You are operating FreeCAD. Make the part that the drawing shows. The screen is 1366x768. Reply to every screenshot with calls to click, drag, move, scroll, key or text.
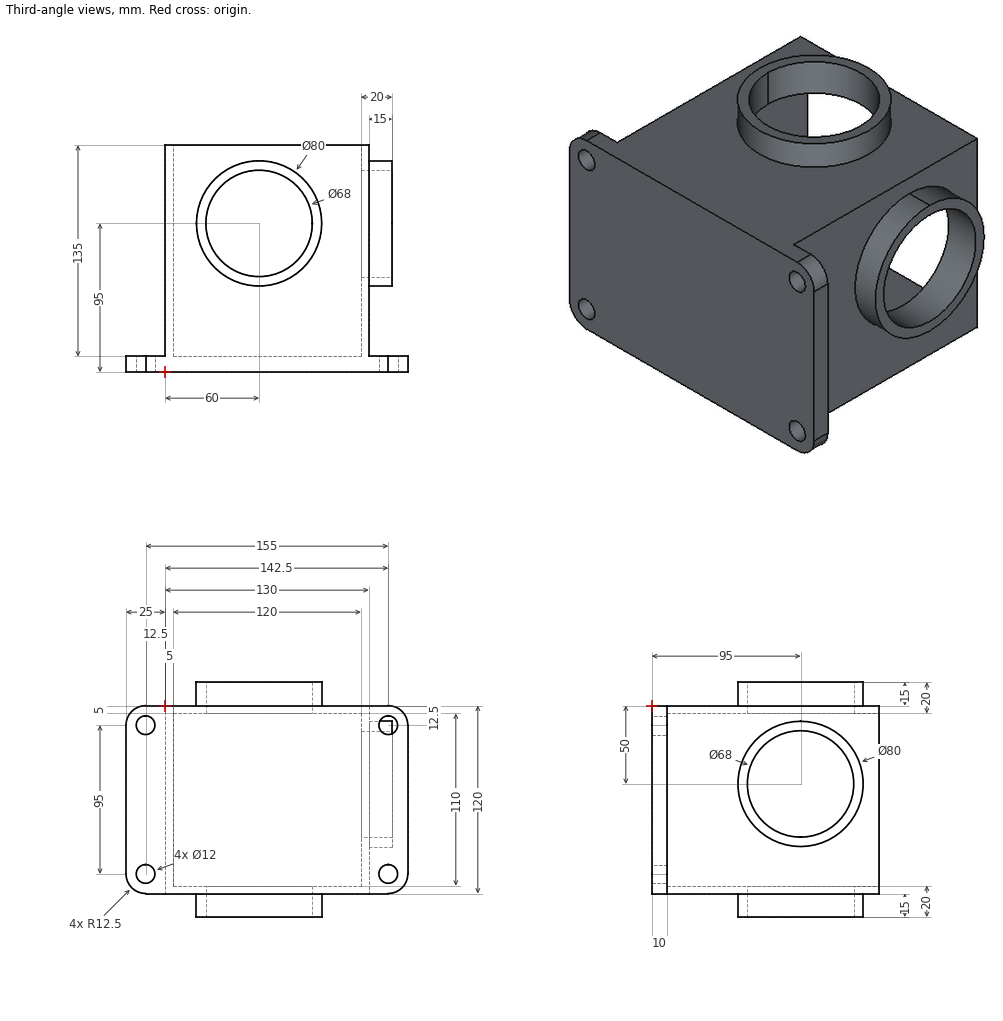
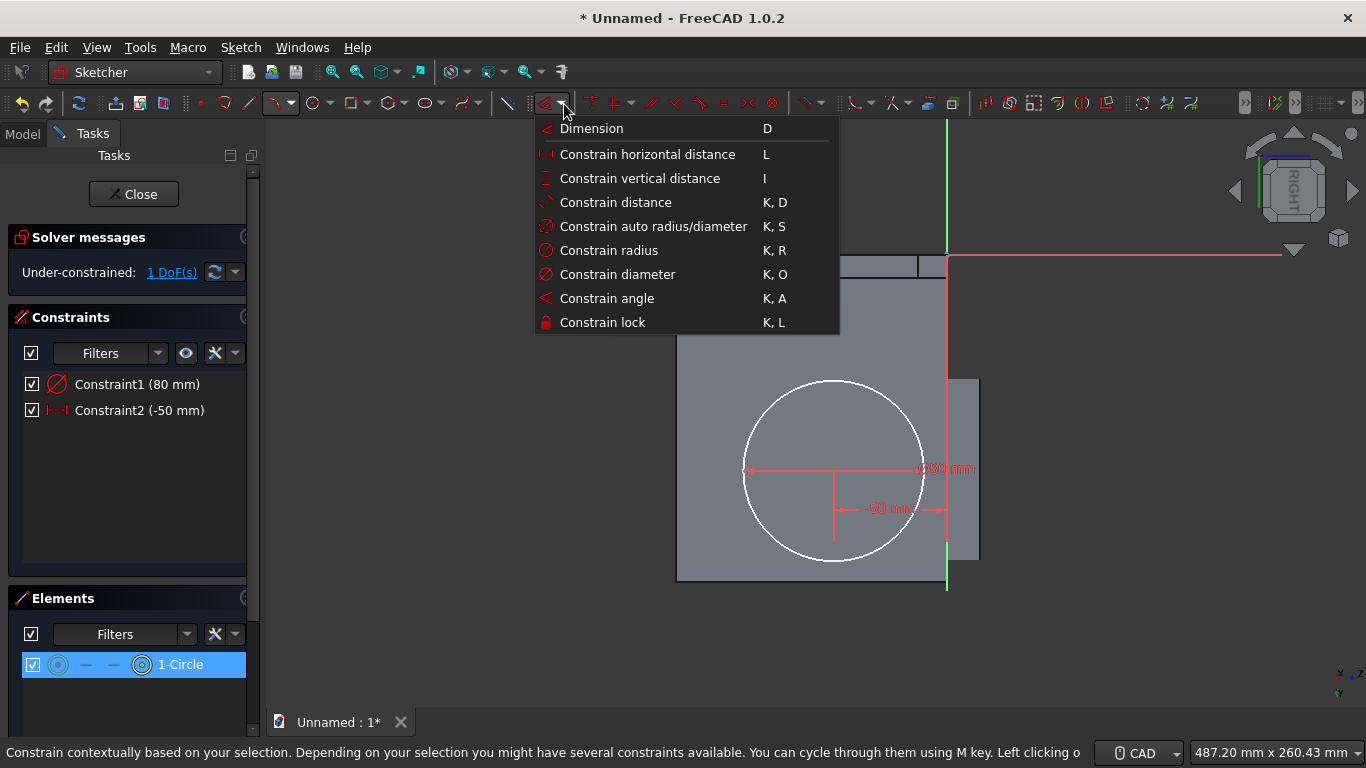
click(687, 178)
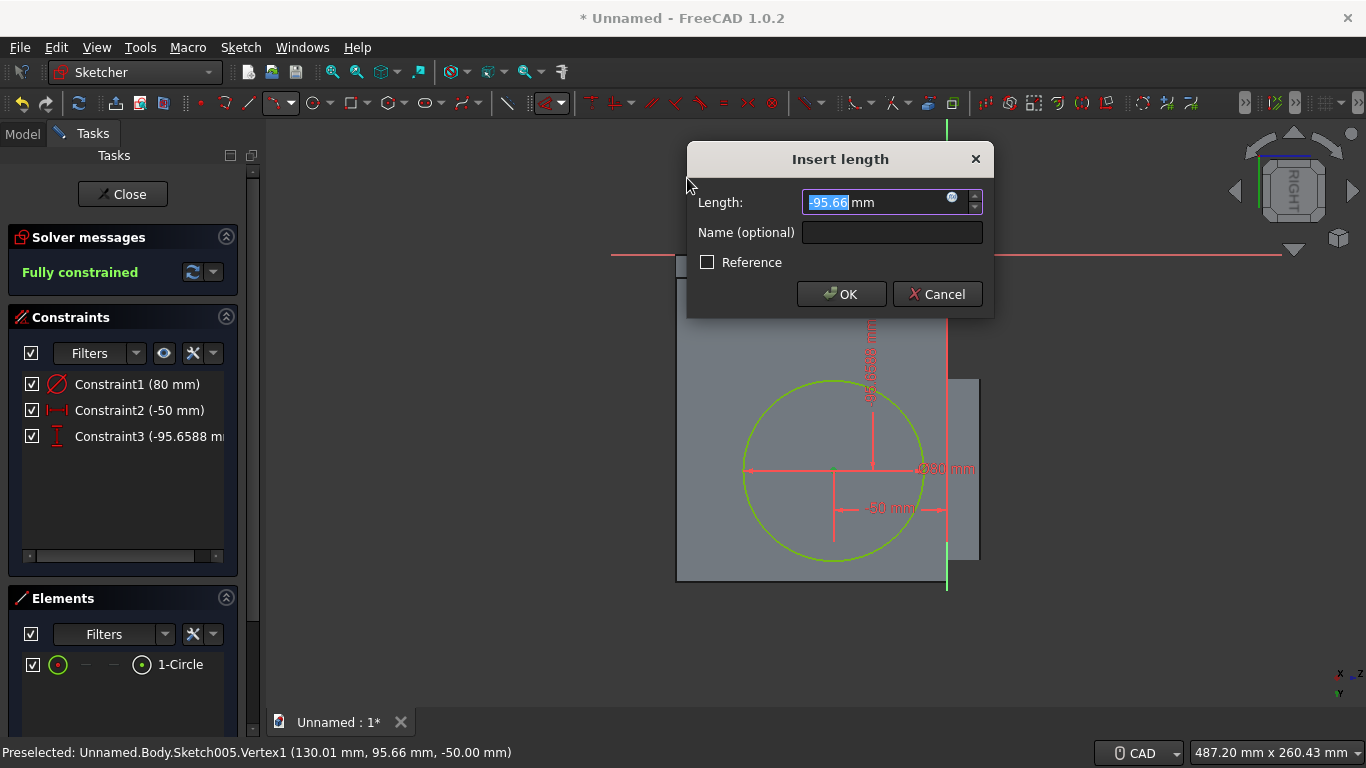
text(-95)
key(Return)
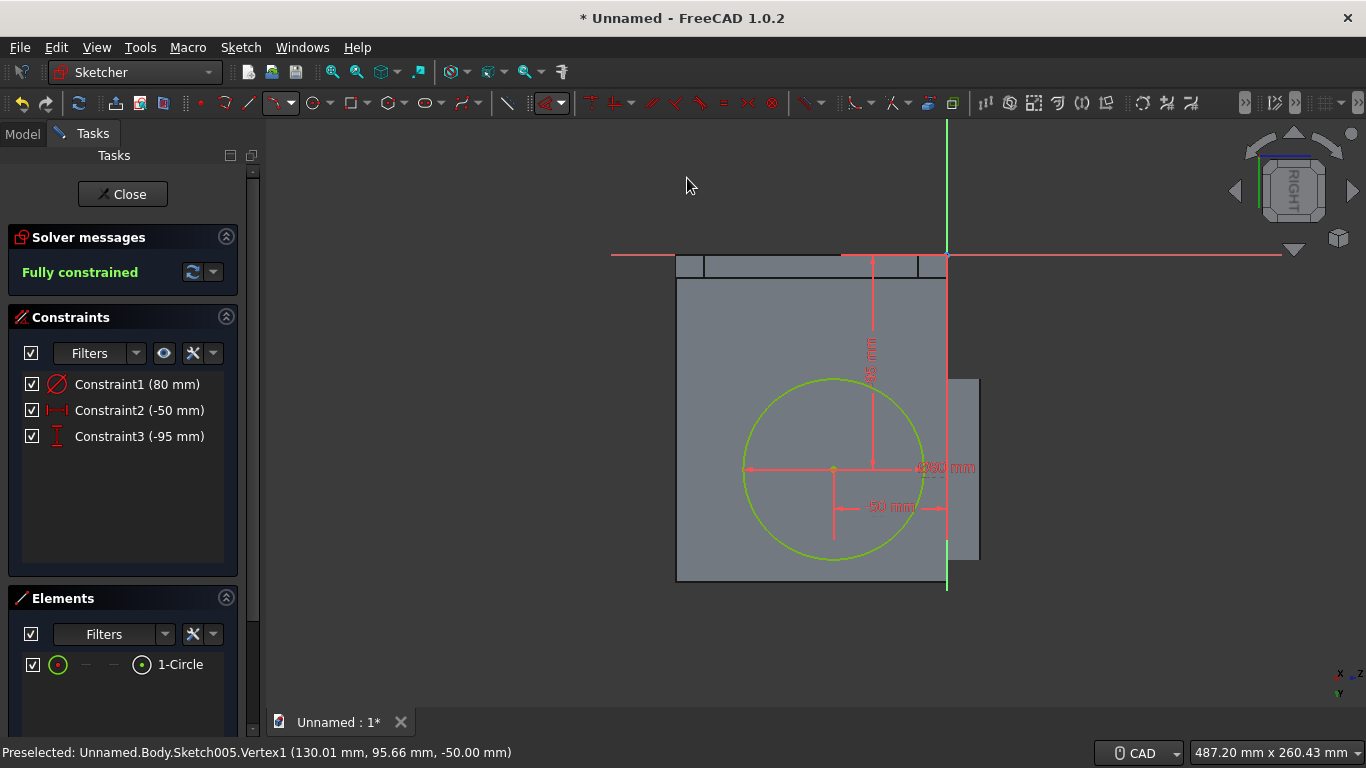
click(123, 194)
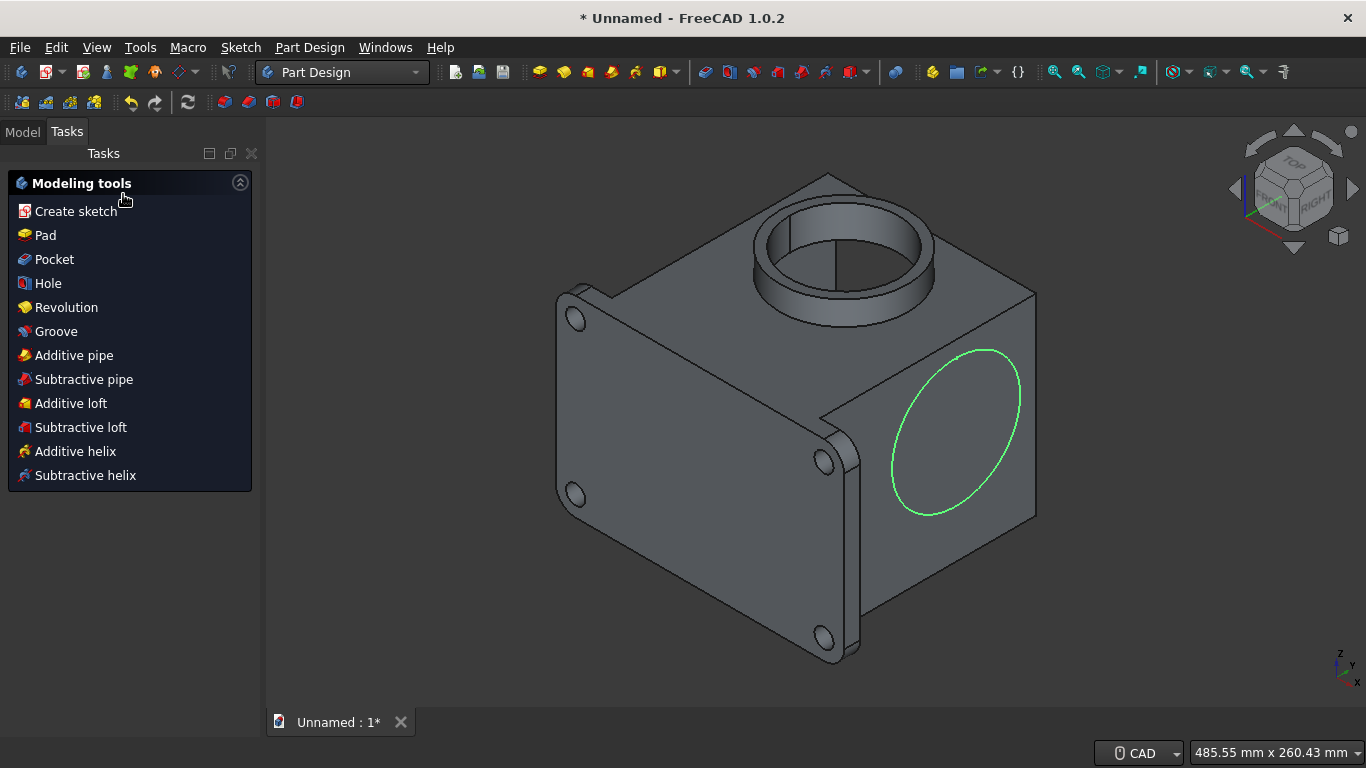
click(540, 72)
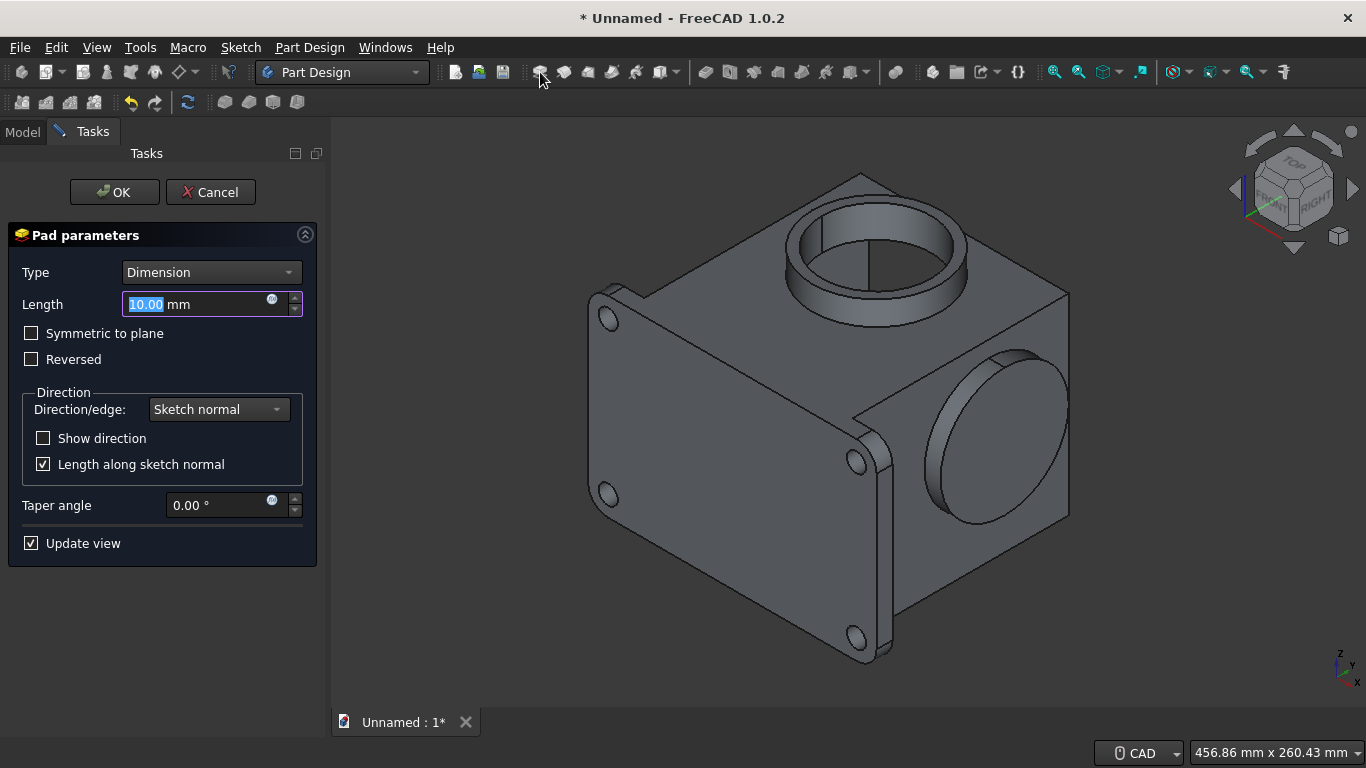
text(15)
key(Tab)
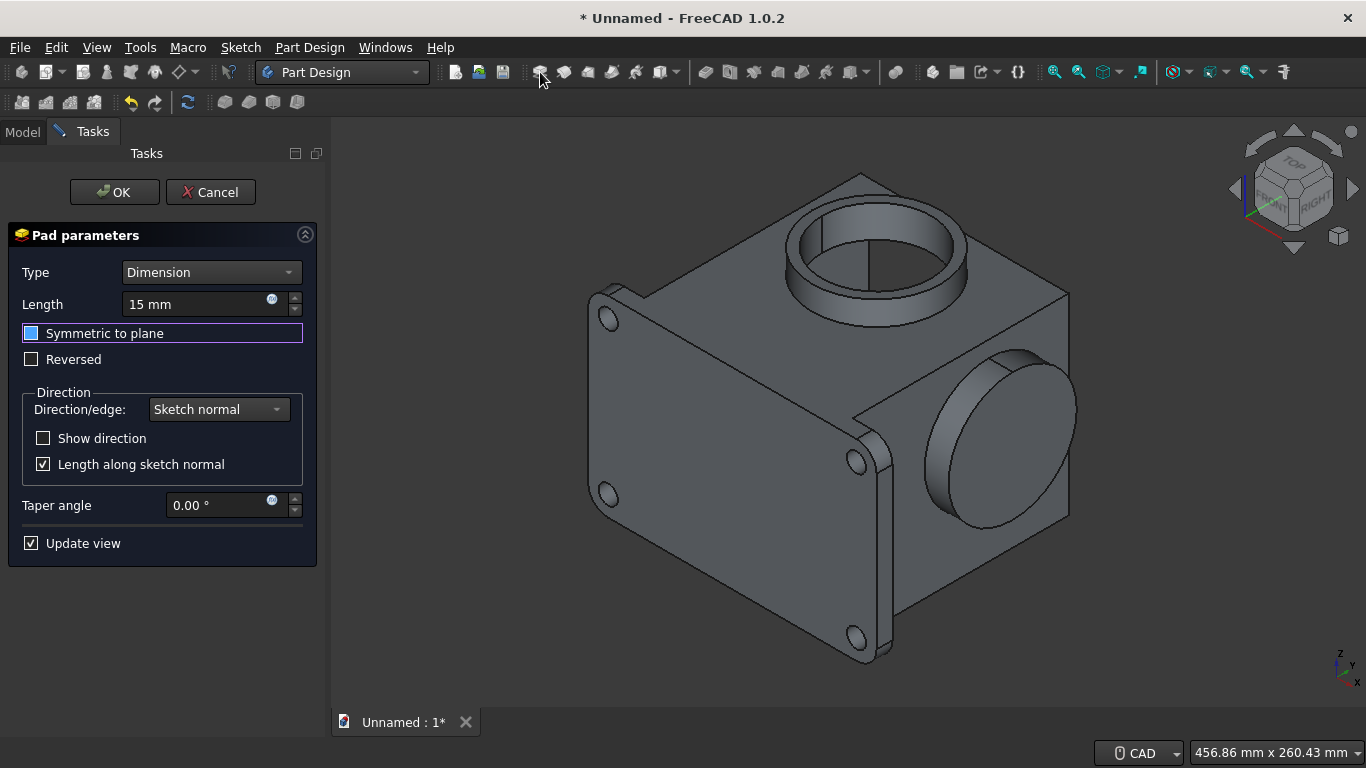
click(115, 192)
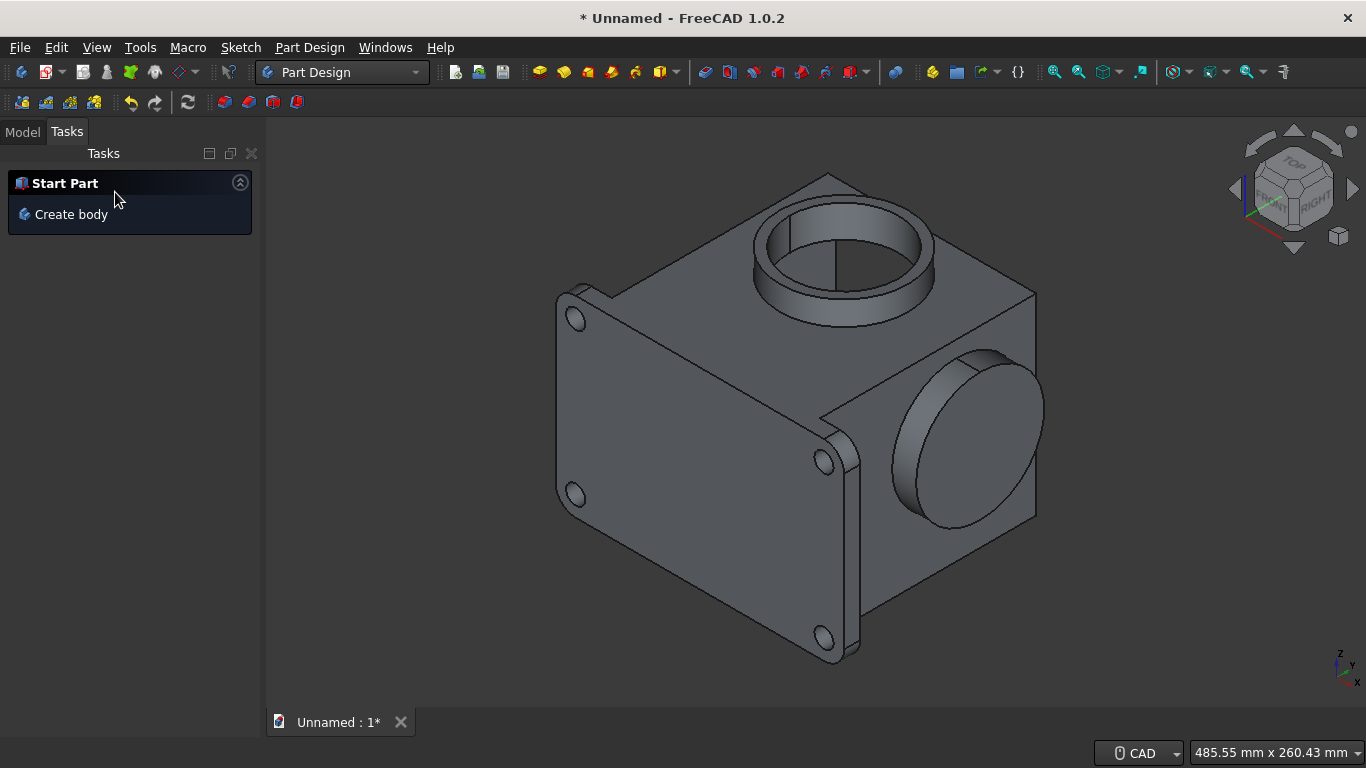
click(980, 445)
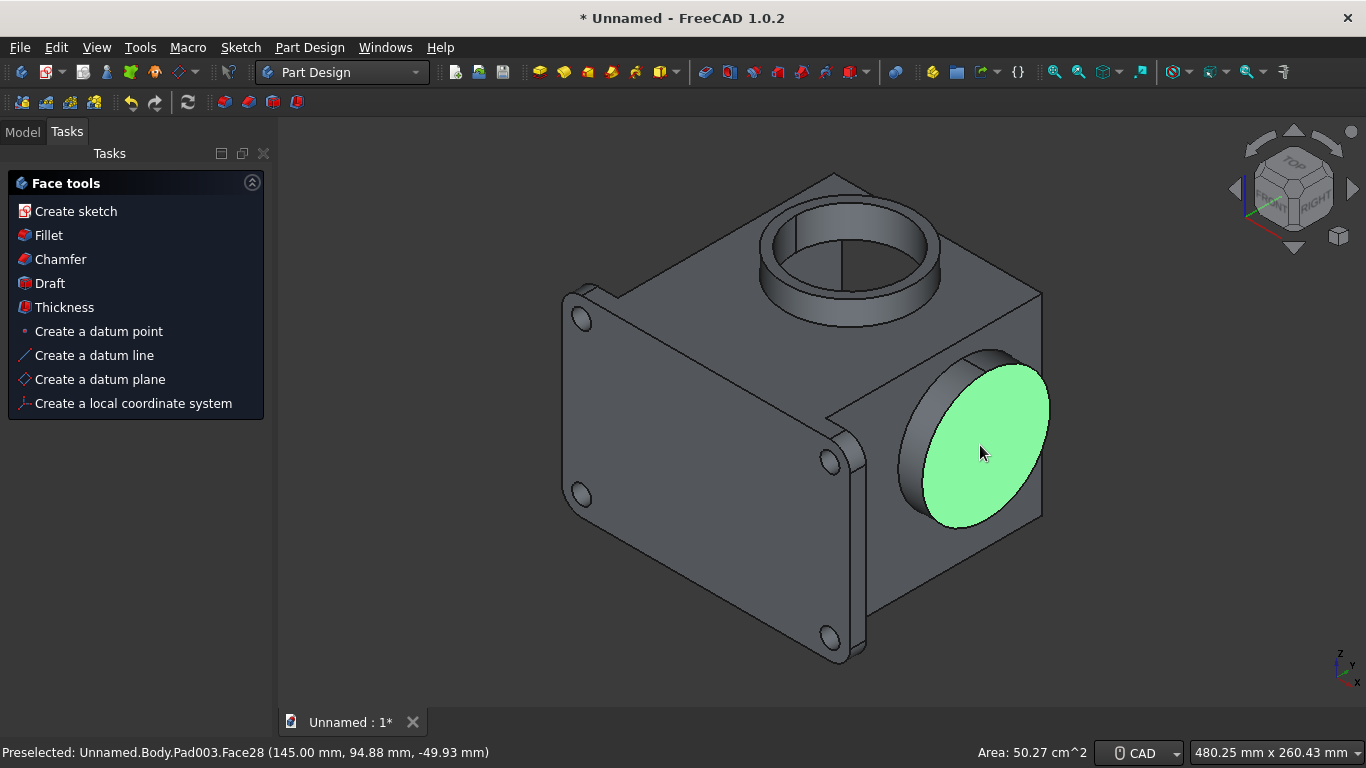
click(46, 72)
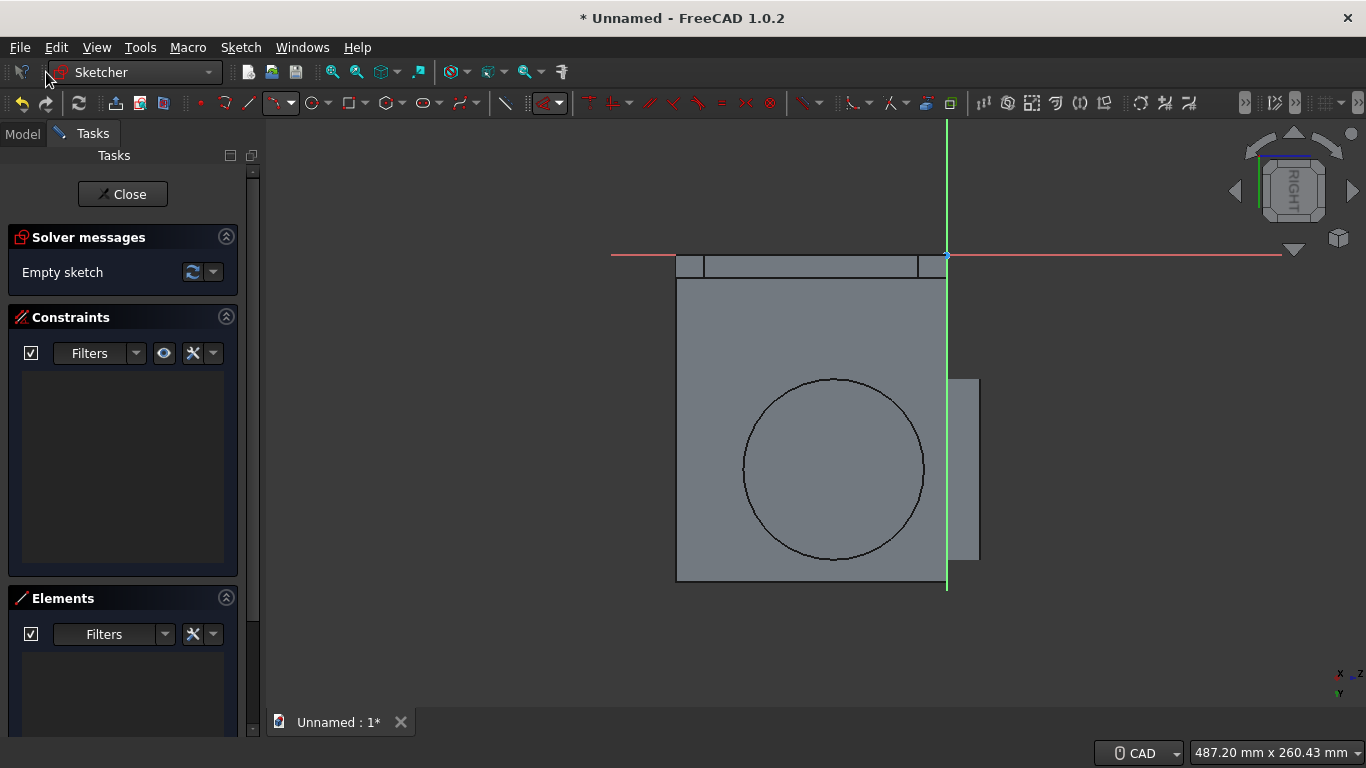
click(164, 104)